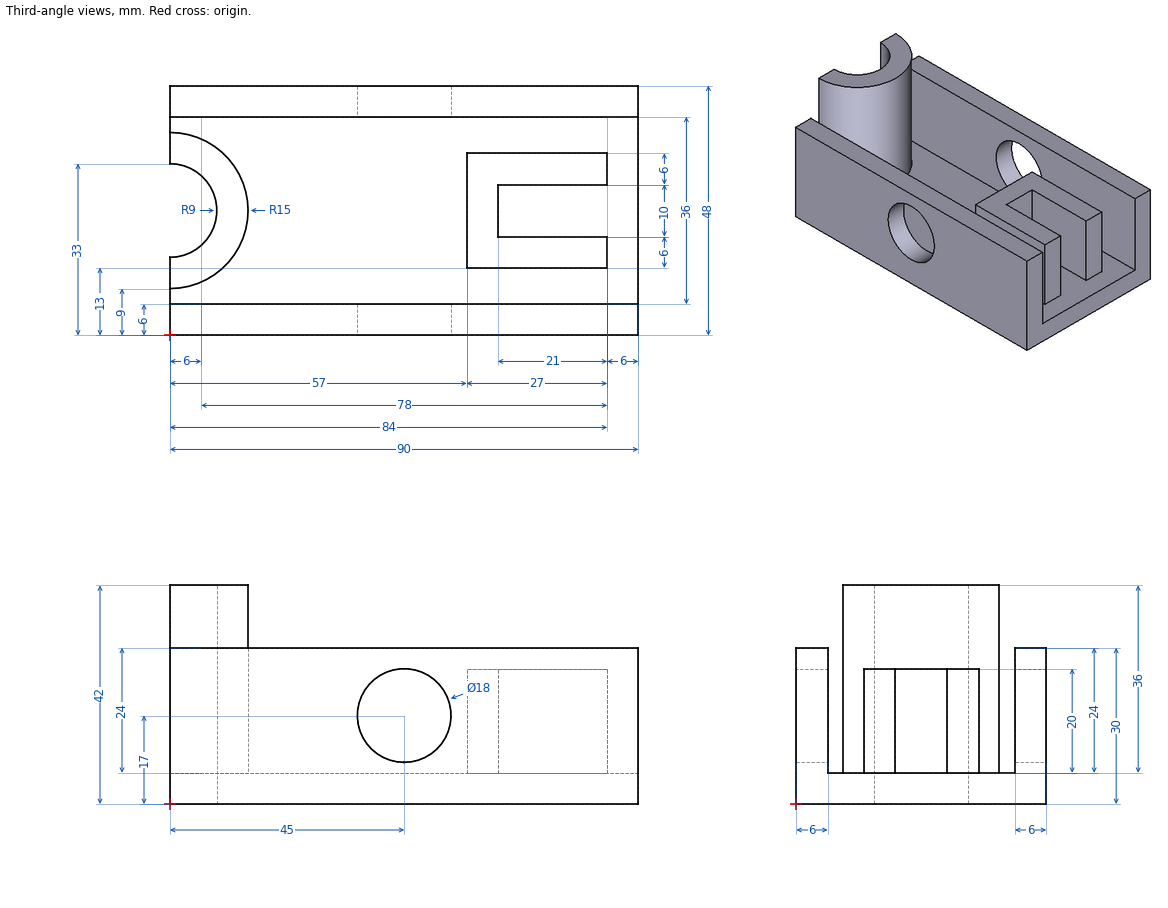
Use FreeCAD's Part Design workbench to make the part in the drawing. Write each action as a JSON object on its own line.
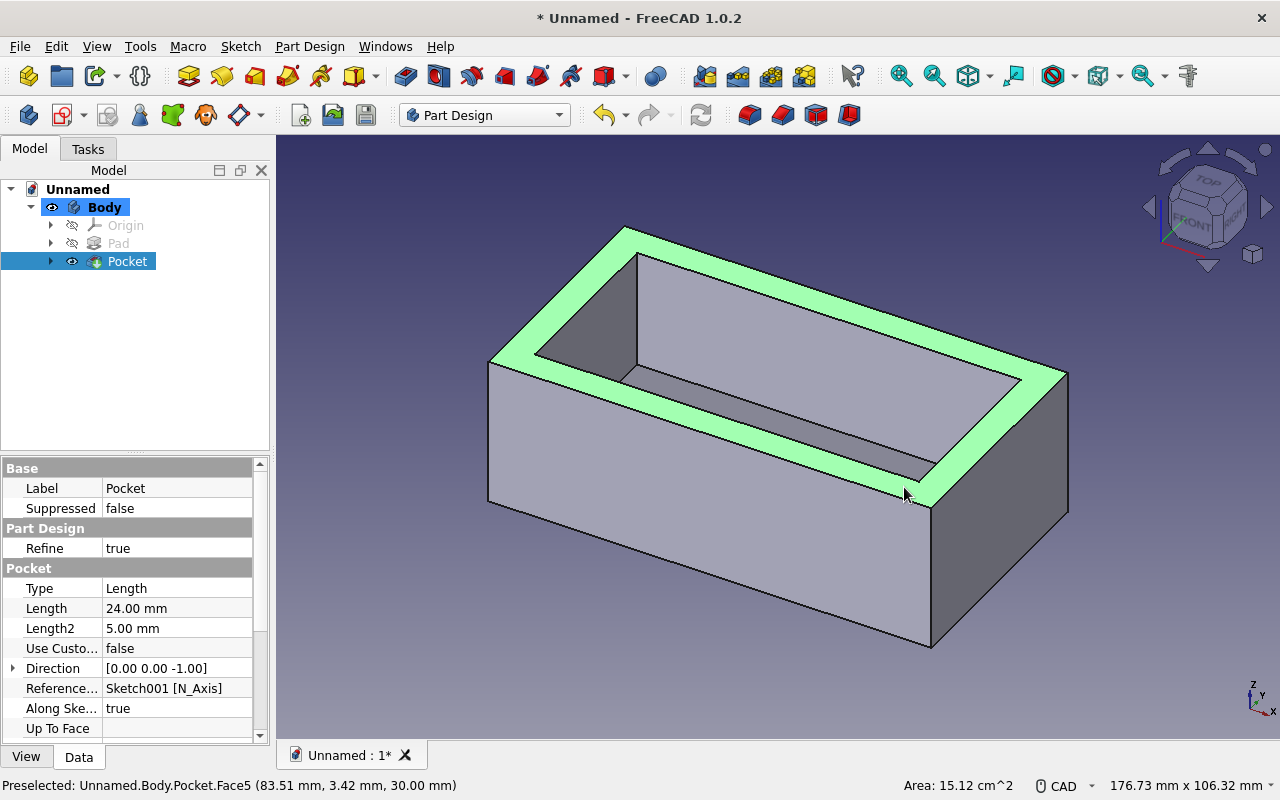
{"action": "left_click", "coordinate": [62, 116]}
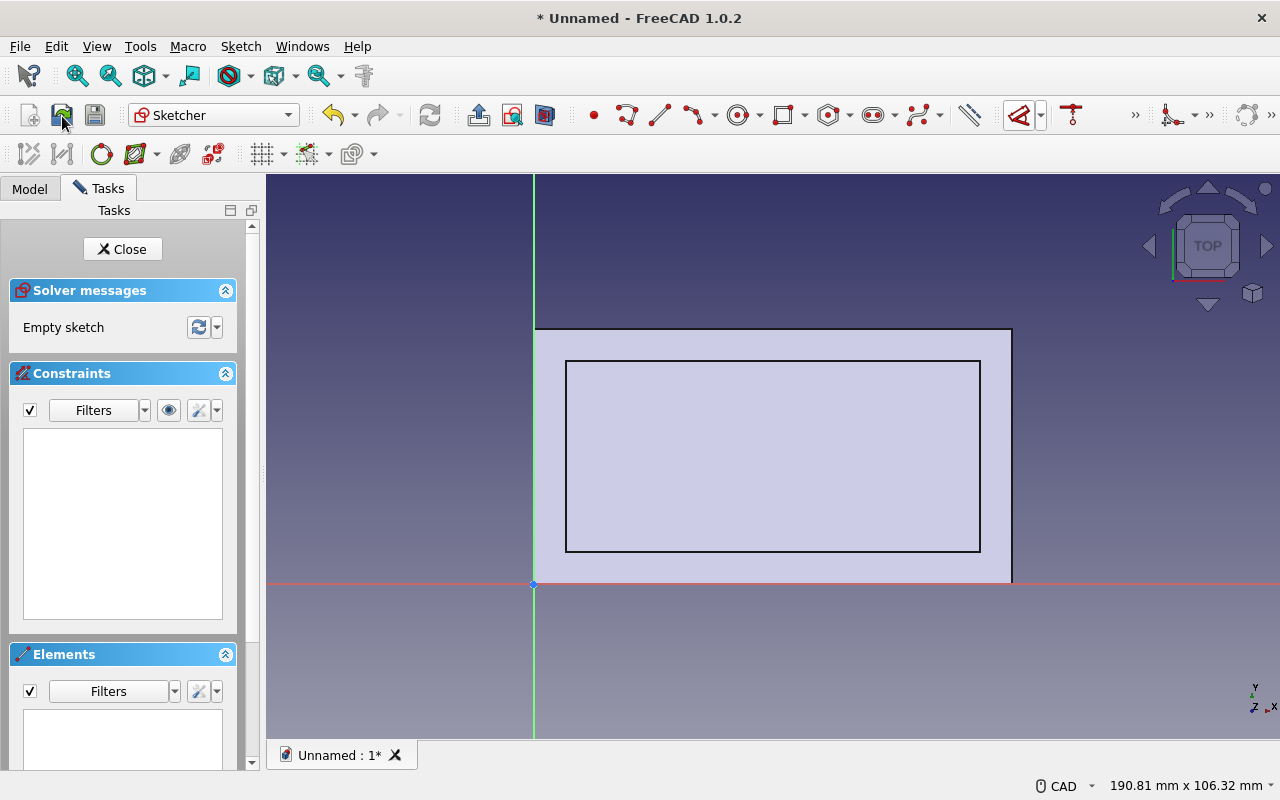
{"action": "scroll", "coordinate": [294, 505], "scroll_direction": "up", "scroll_amount": 2}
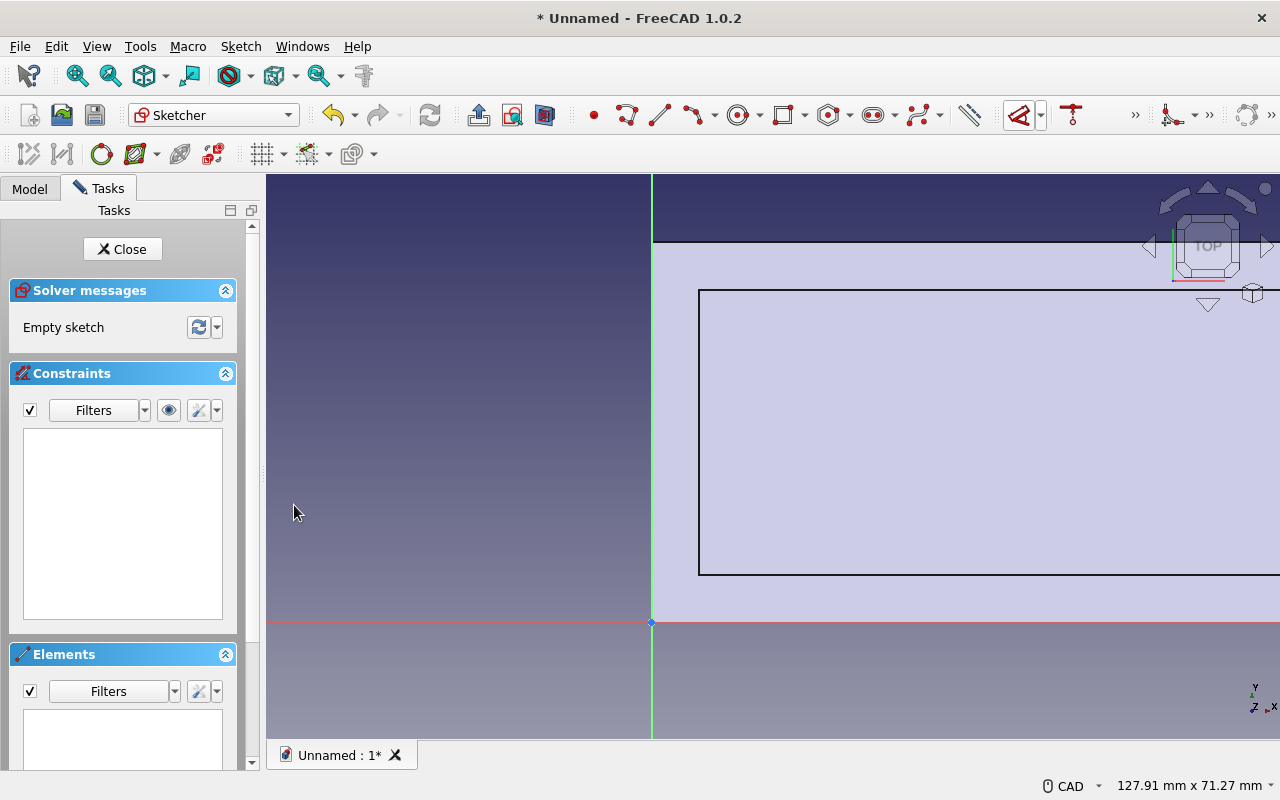
{"action": "key", "text": "g r"}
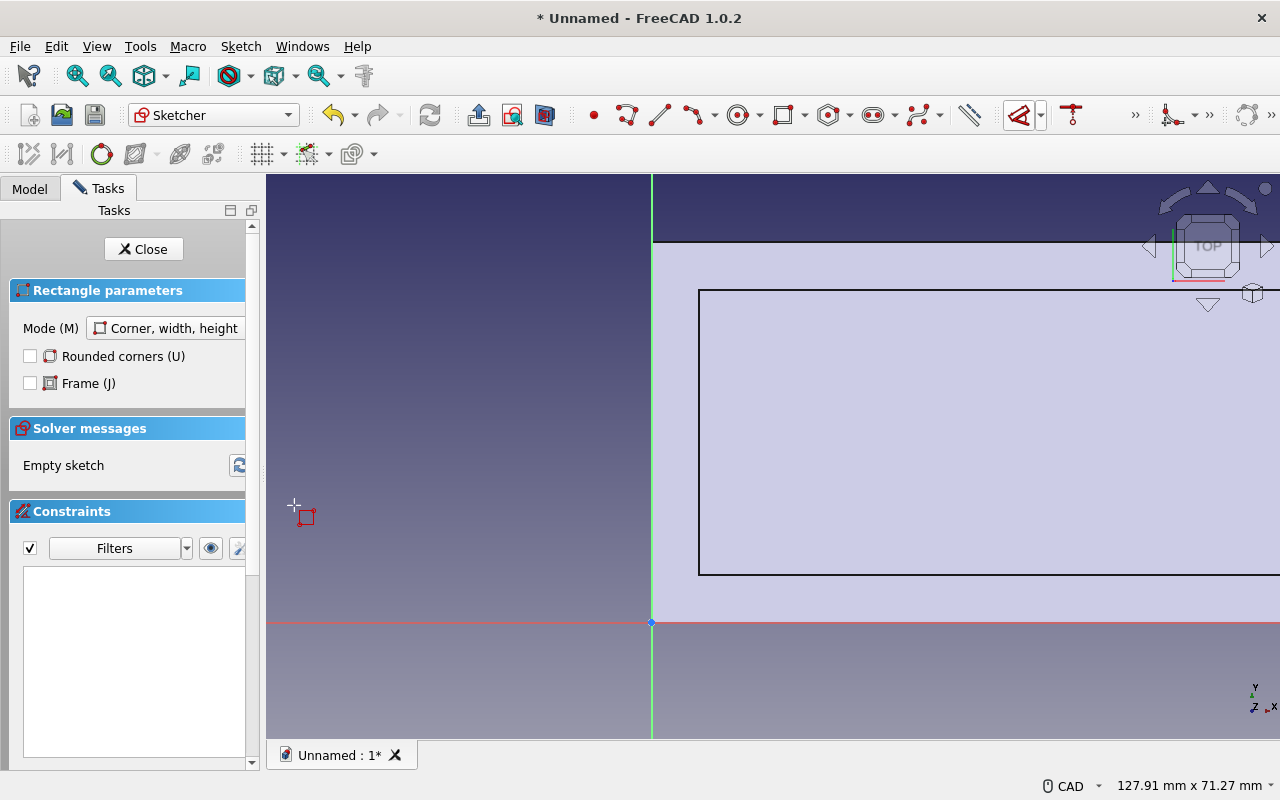
{"action": "left_click", "coordinate": [652, 290]}
{"action": "mouse_move", "coordinate": [699, 575]}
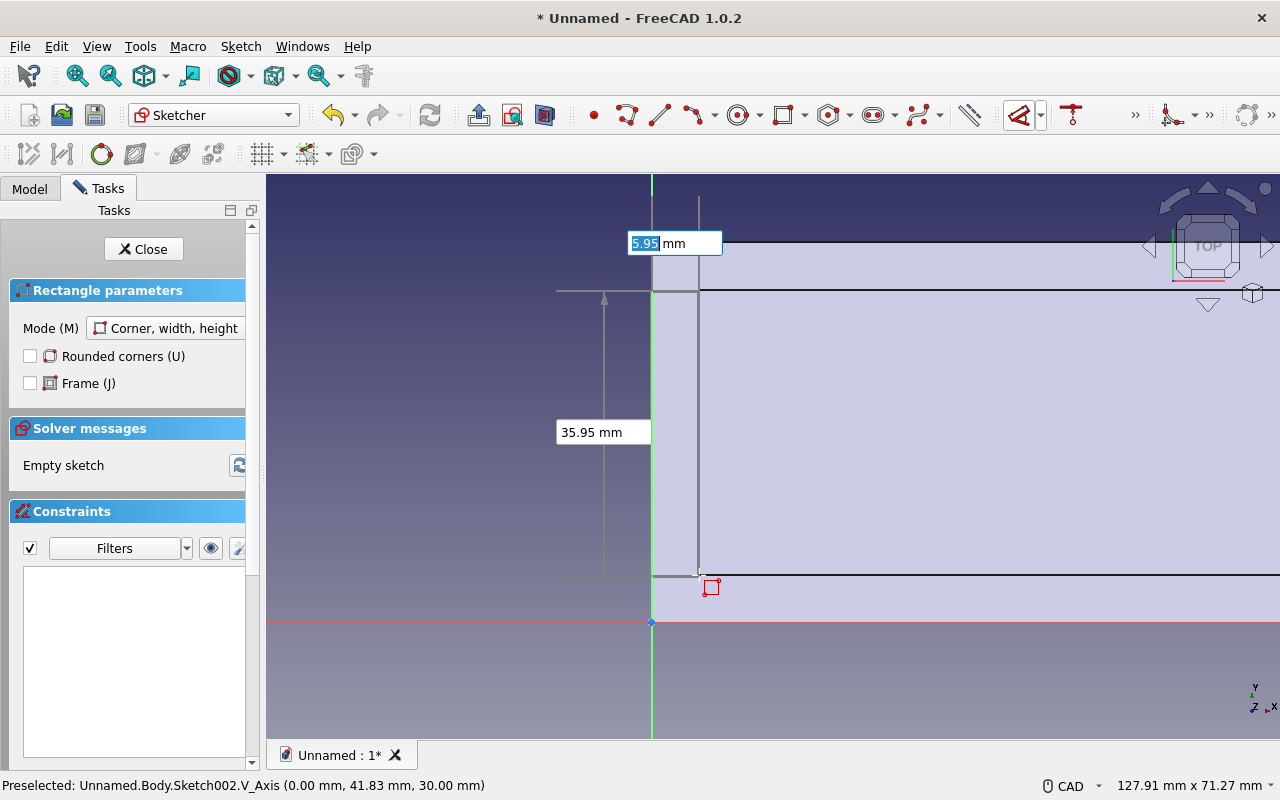
{"action": "type", "text": "6"}
{"action": "key", "text": "Tab"}
{"action": "type", "text": "36"}
{"action": "key", "text": "Return"}
{"action": "key", "text": "Escape"}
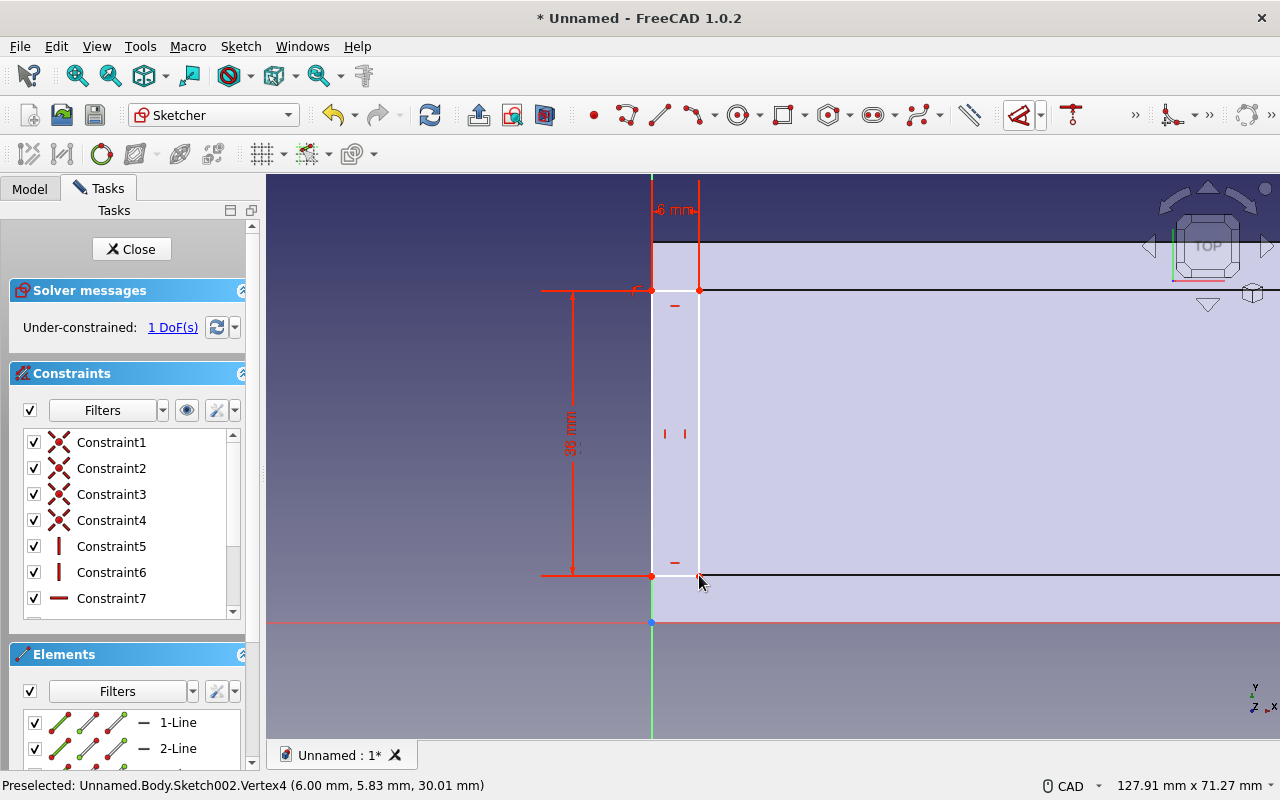
{"action": "left_click", "coordinate": [1018, 116]}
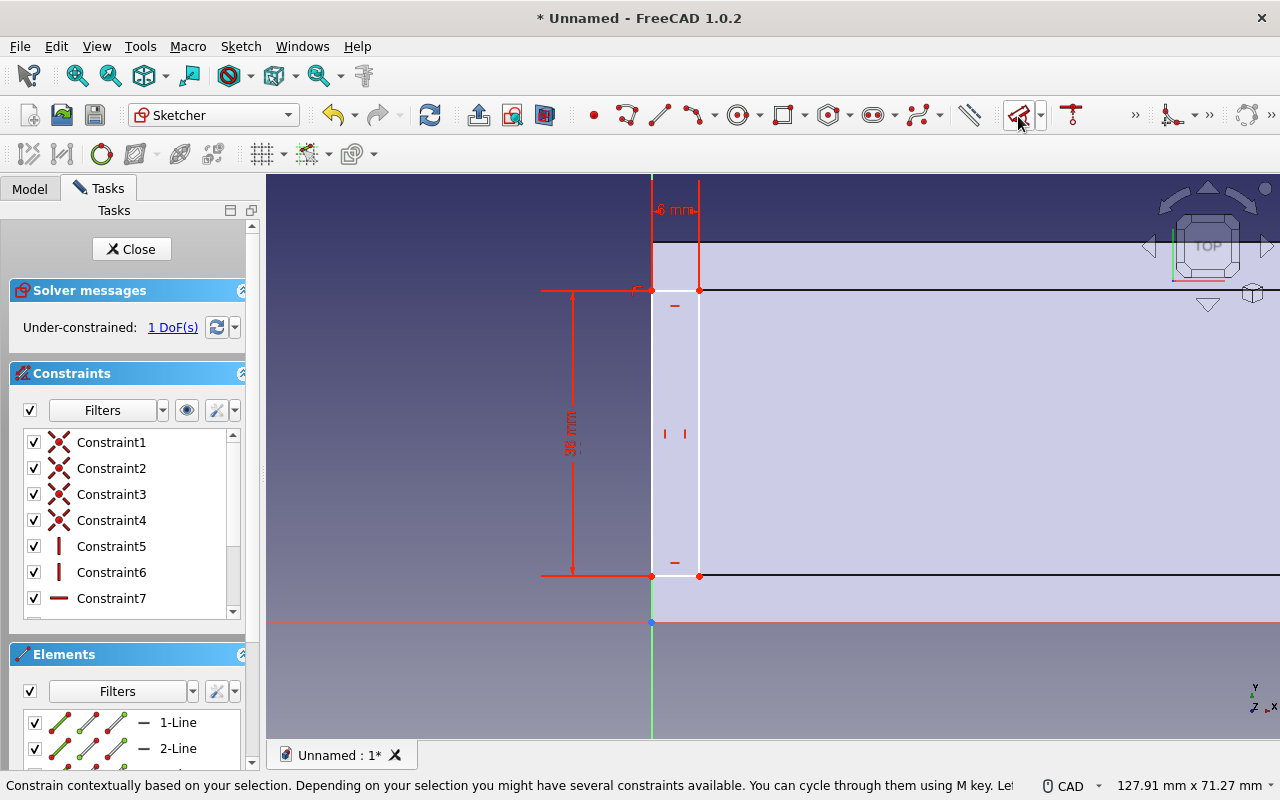
{"action": "left_click", "coordinate": [652, 576]}
{"action": "left_click", "coordinate": [618, 600]}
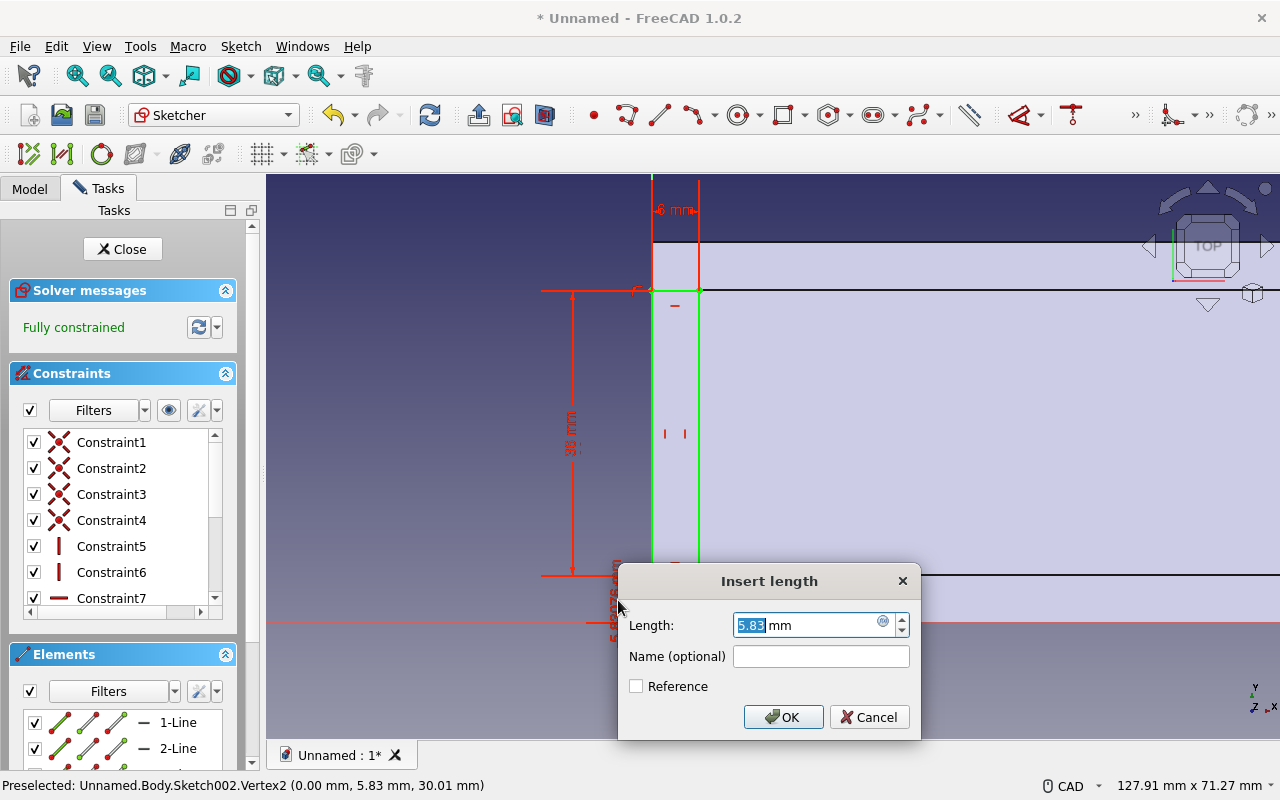
{"action": "type", "text": "6"}
{"action": "key", "text": "Return"}
{"action": "key", "text": "Escape"}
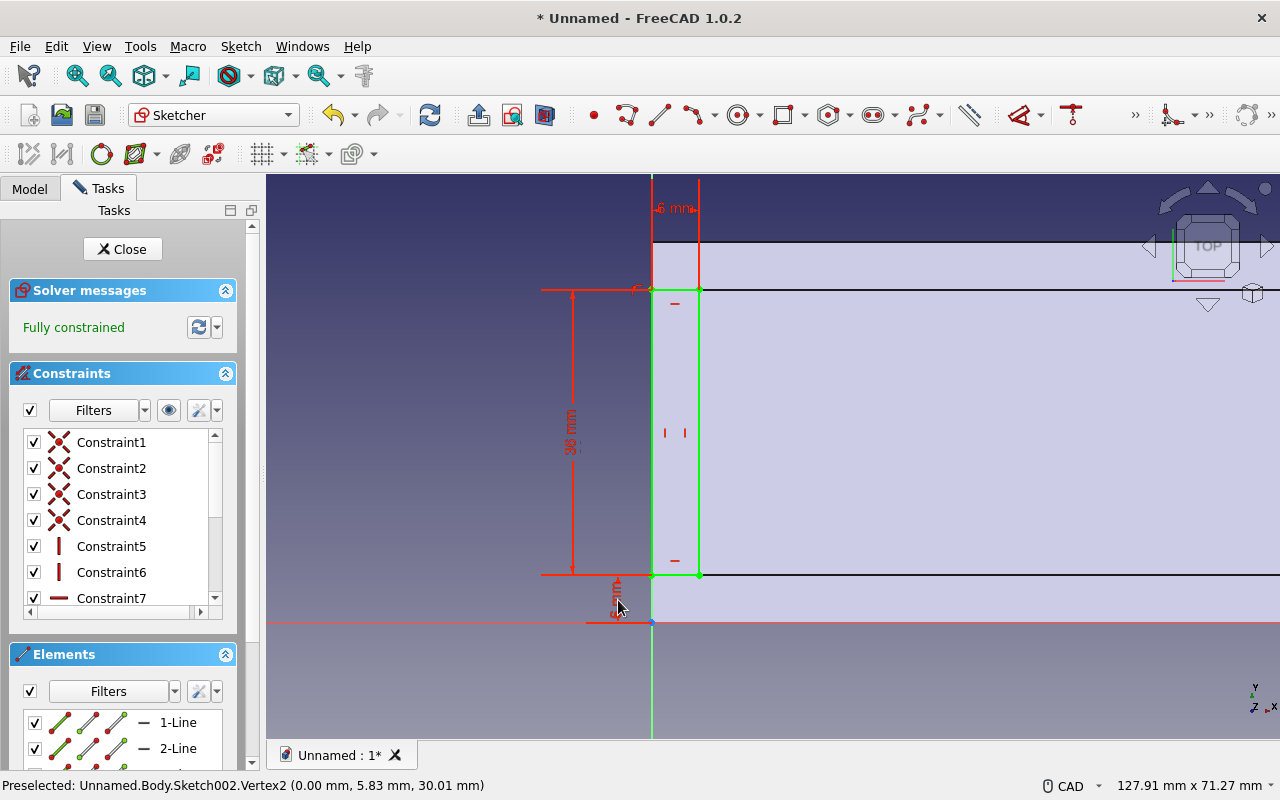
{"action": "left_click", "coordinate": [123, 249]}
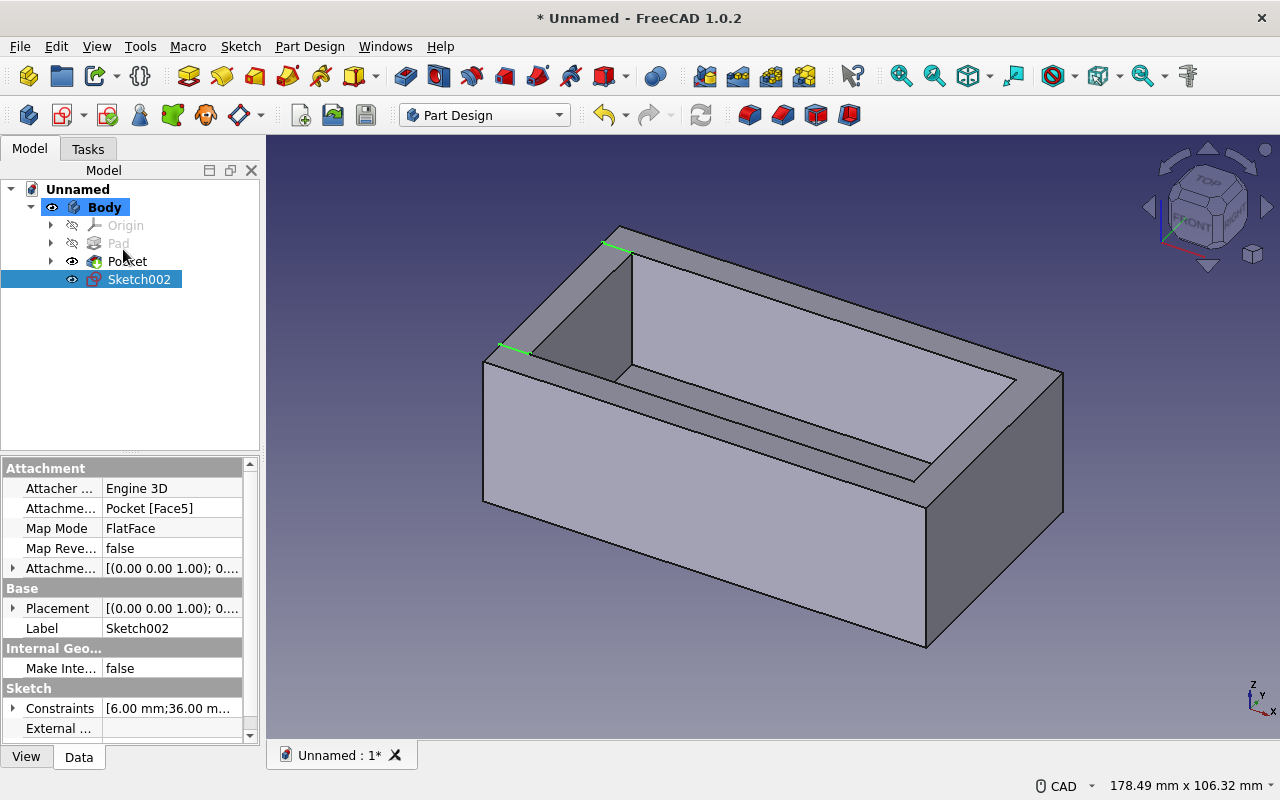
{"action": "left_click", "coordinate": [406, 76]}